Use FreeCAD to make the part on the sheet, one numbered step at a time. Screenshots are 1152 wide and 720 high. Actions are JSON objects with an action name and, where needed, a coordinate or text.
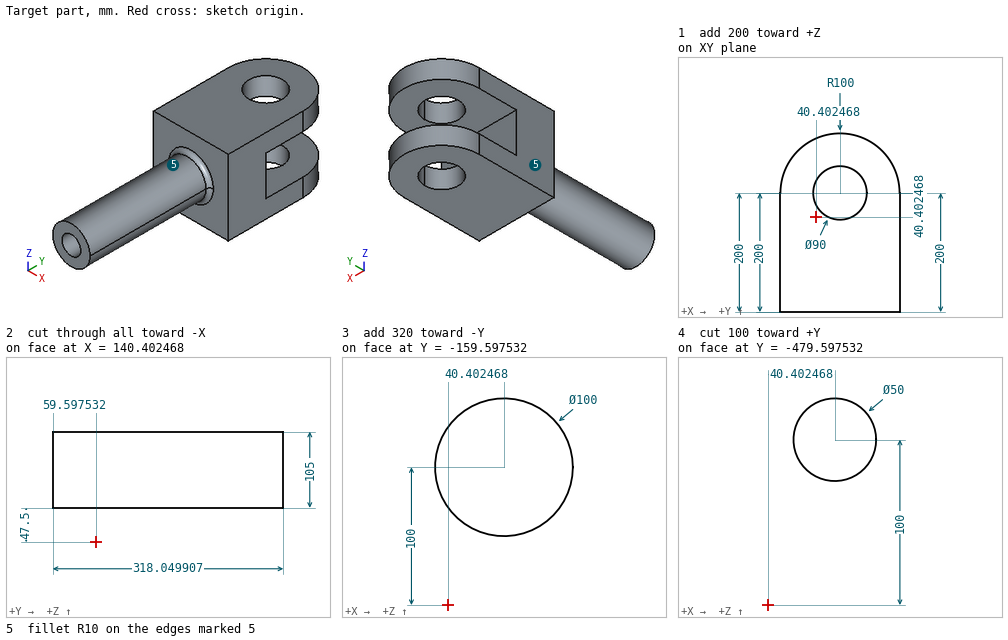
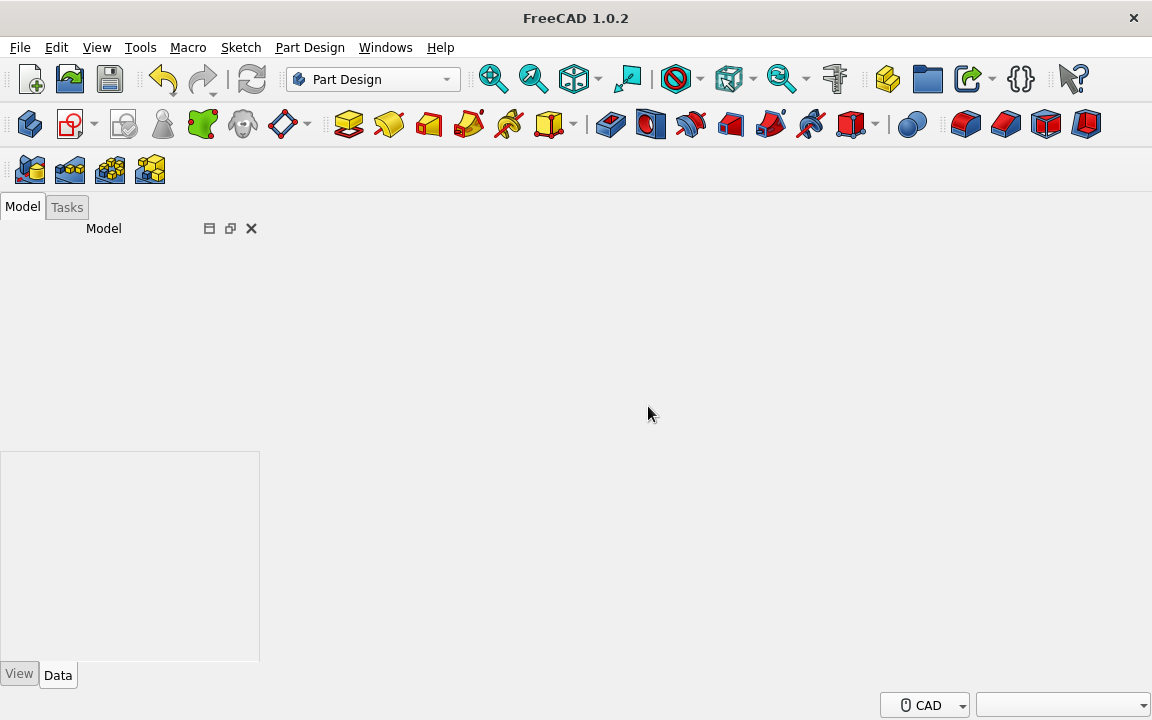
{"action": "key", "text": "ctrl+n"}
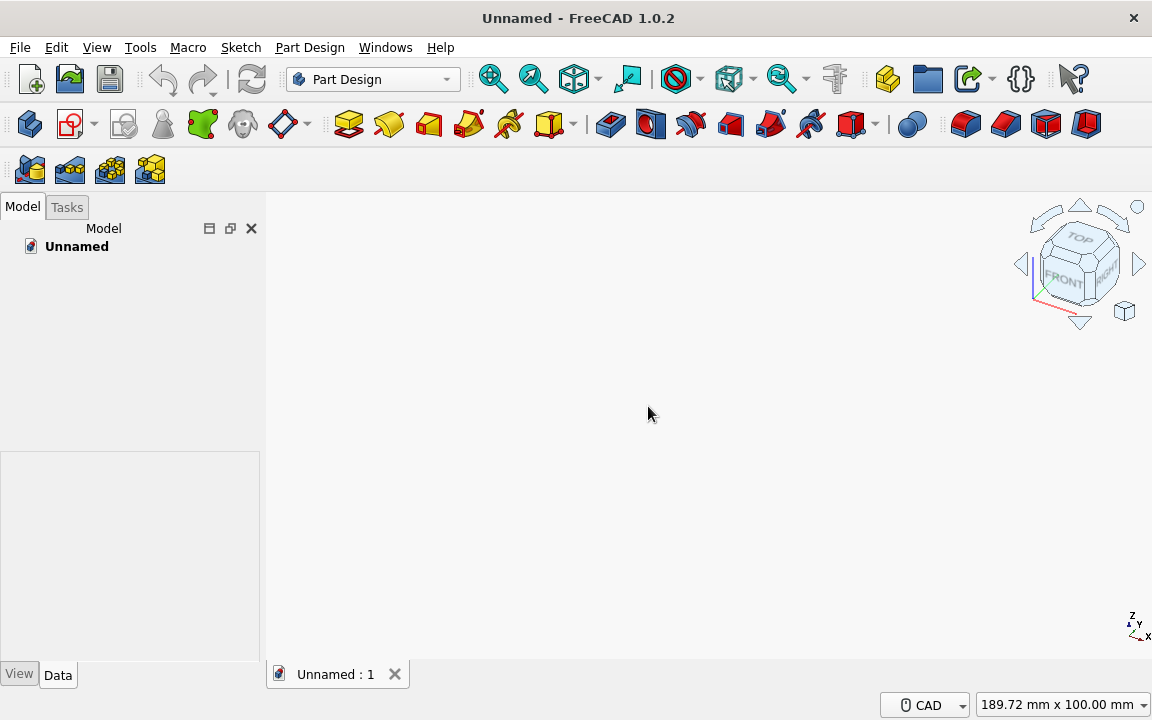
{"action": "left_click", "coordinate": [70, 124]}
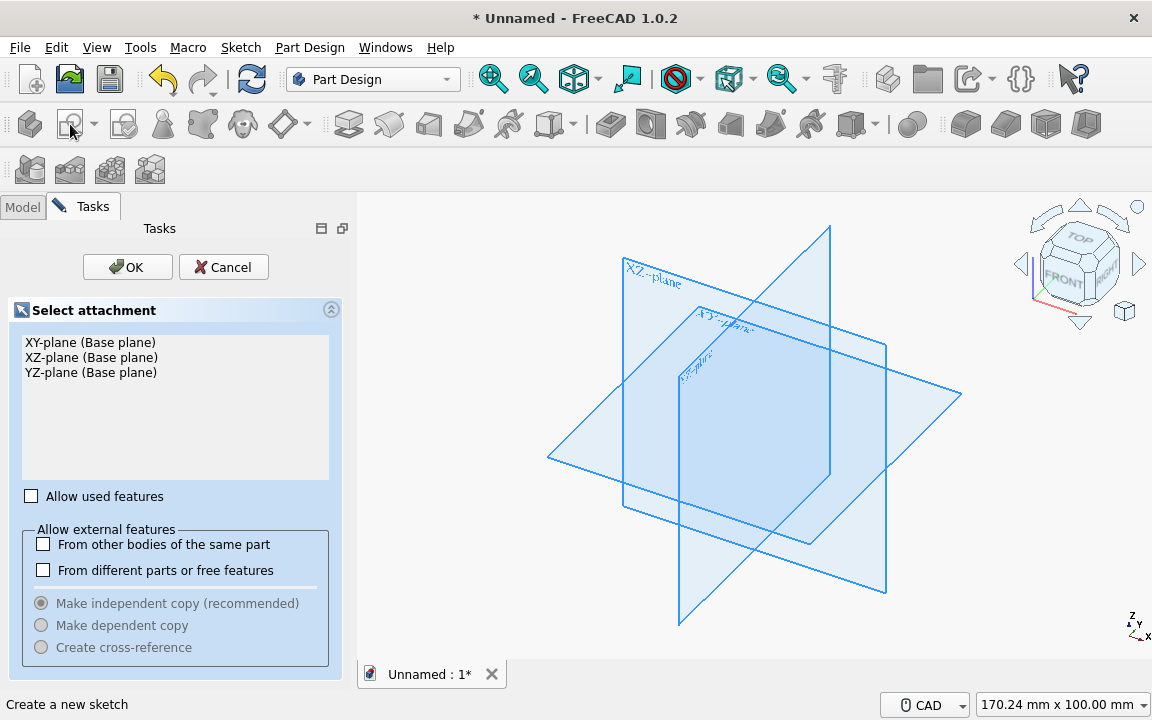
{"action": "left_click", "coordinate": [82, 342]}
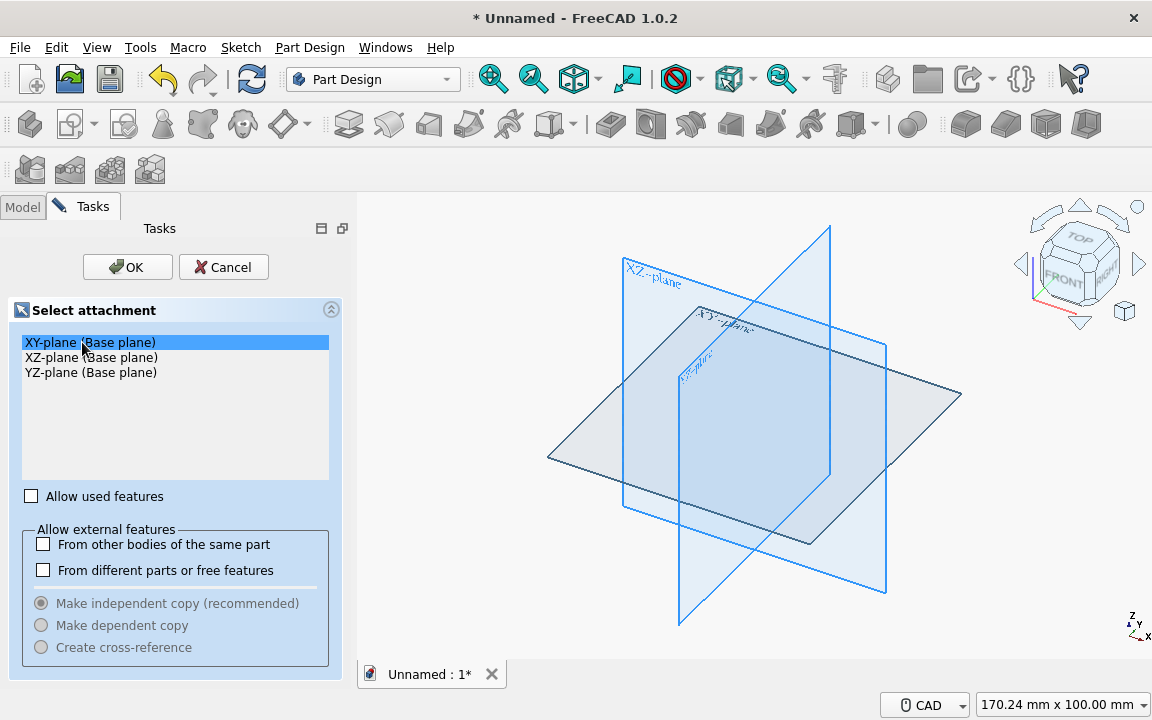
{"action": "left_click", "coordinate": [128, 267]}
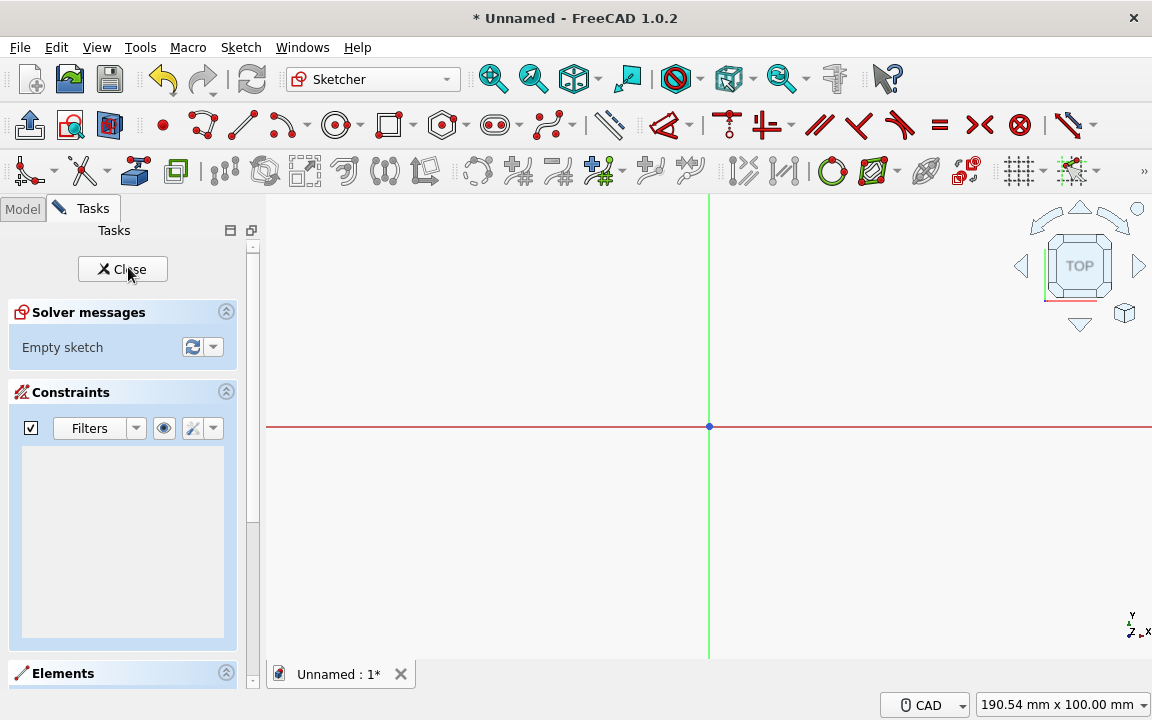
{"action": "scroll", "coordinate": [576, 415], "scroll_direction": "down", "scroll_amount": 8}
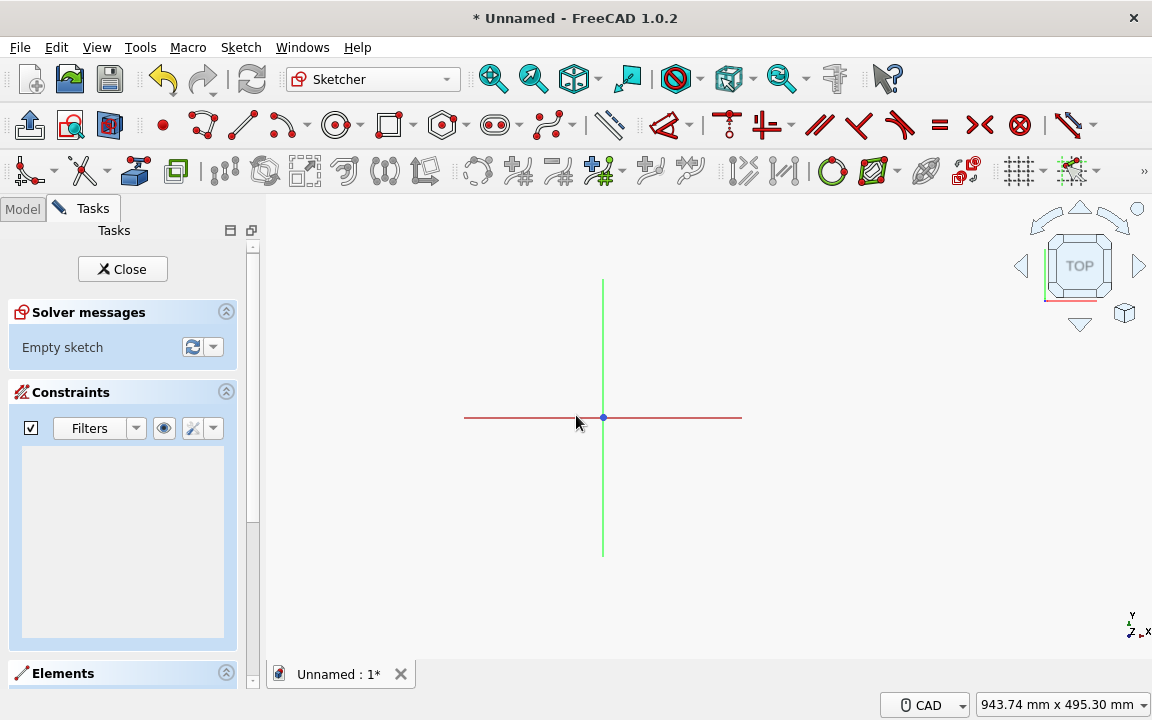
{"action": "key", "text": "g m"}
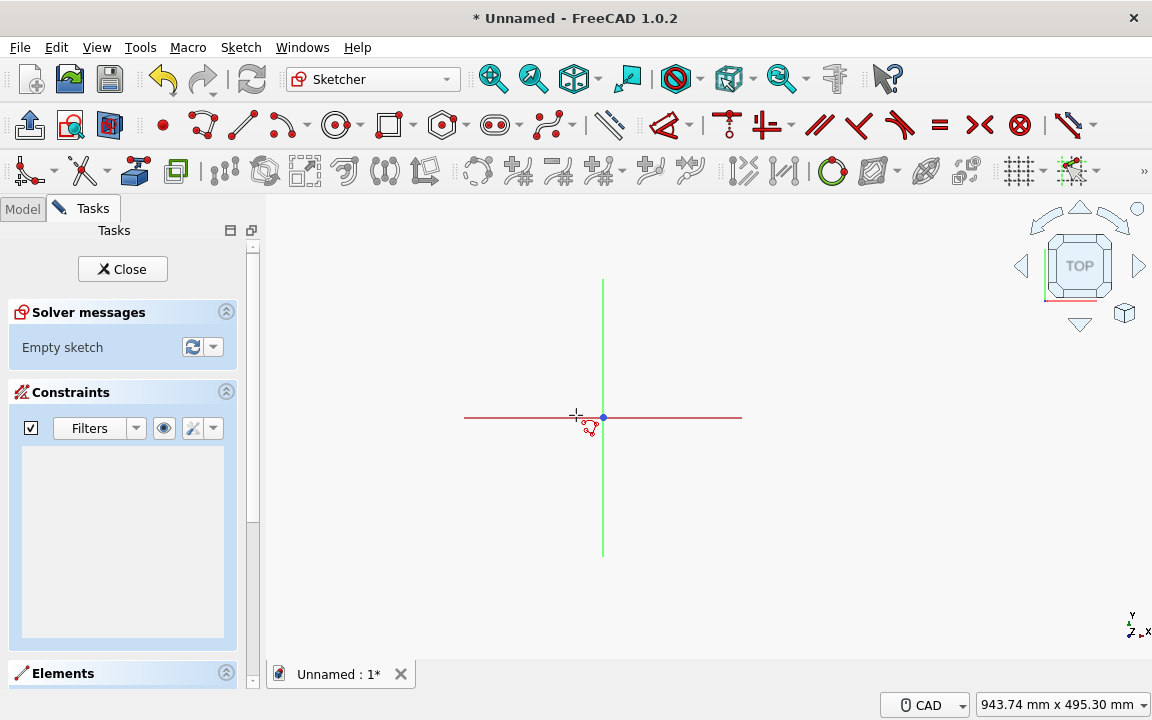
{"action": "left_click", "coordinate": [547, 380]}
{"action": "left_click", "coordinate": [547, 568]}
{"action": "left_click", "coordinate": [735, 568]}
{"action": "left_click", "coordinate": [735, 380]}
{"action": "right_click", "coordinate": [735, 380]}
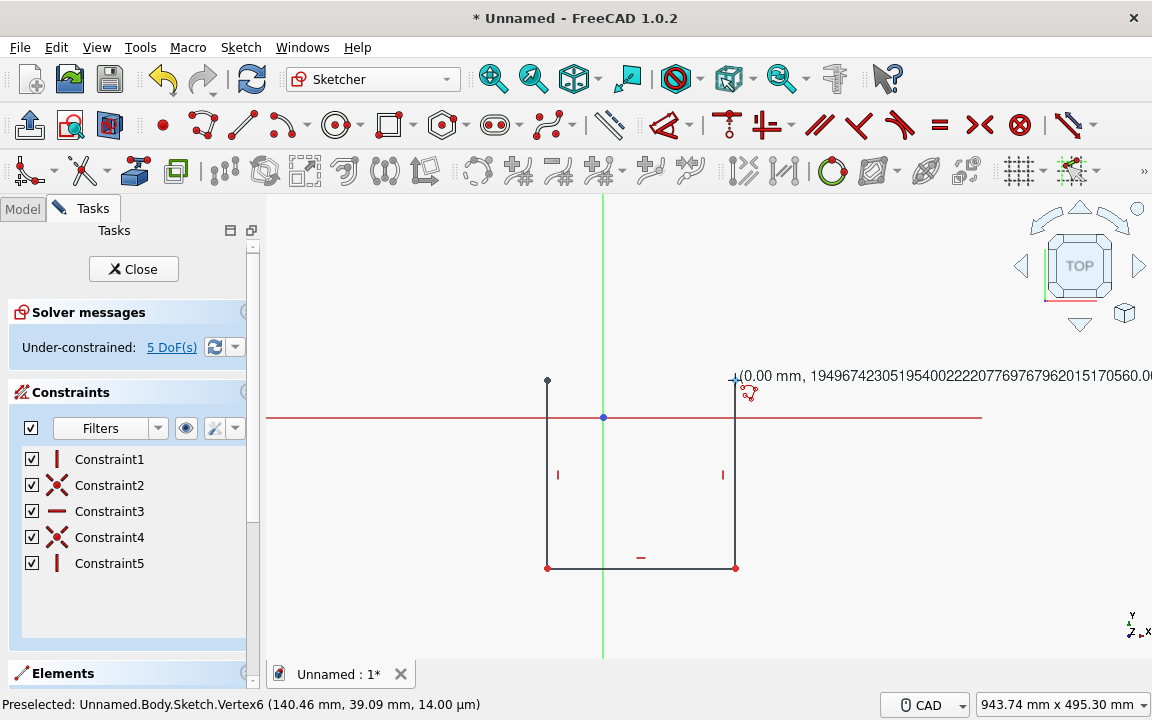
{"action": "key", "text": "g 3 a"}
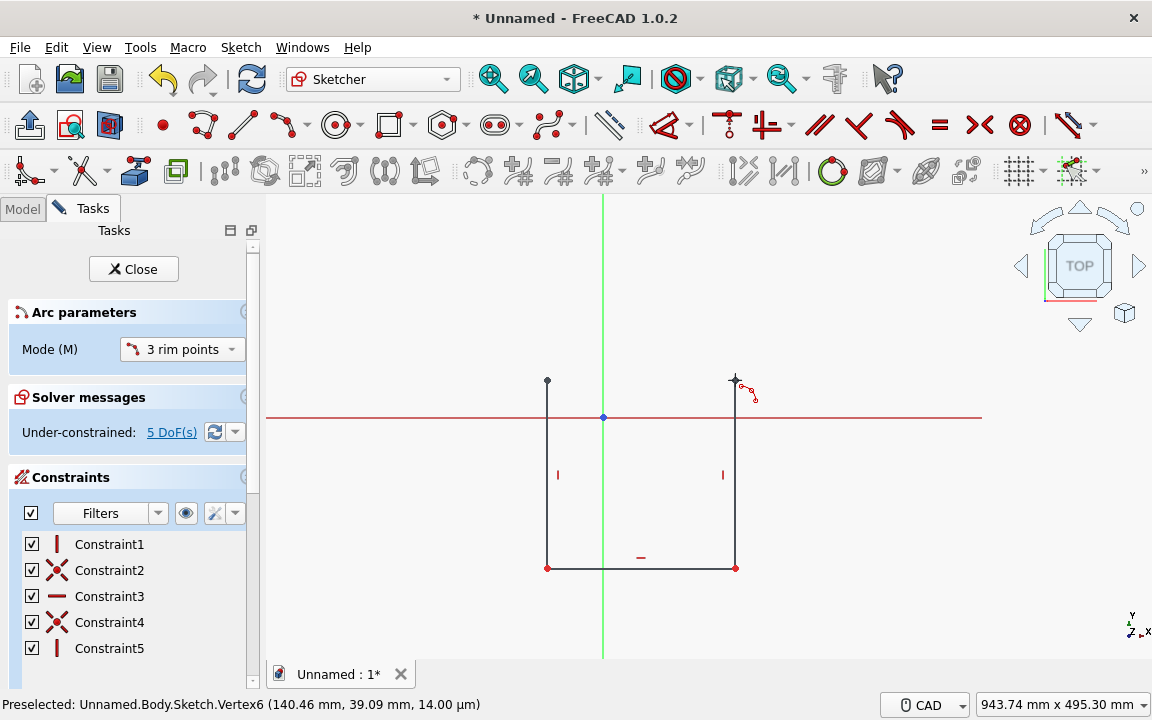
{"action": "left_click", "coordinate": [735, 381]}
{"action": "left_click", "coordinate": [547, 381]}
{"action": "left_click", "coordinate": [641, 286]}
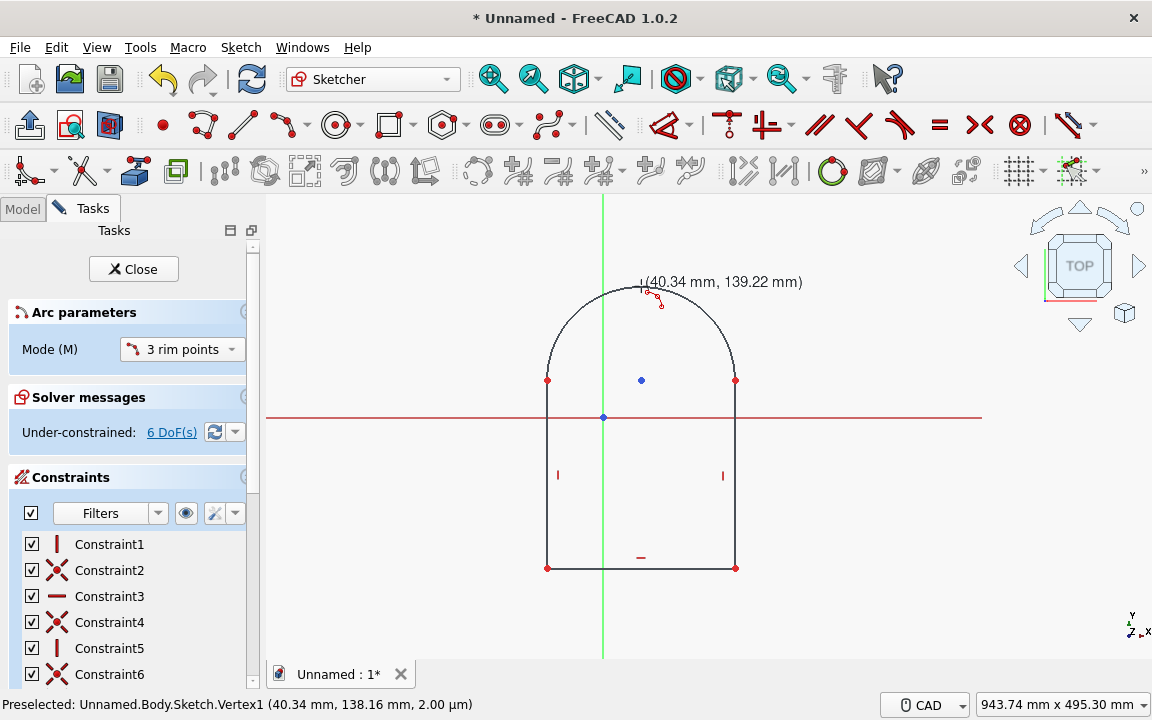
{"action": "key", "text": "g c"}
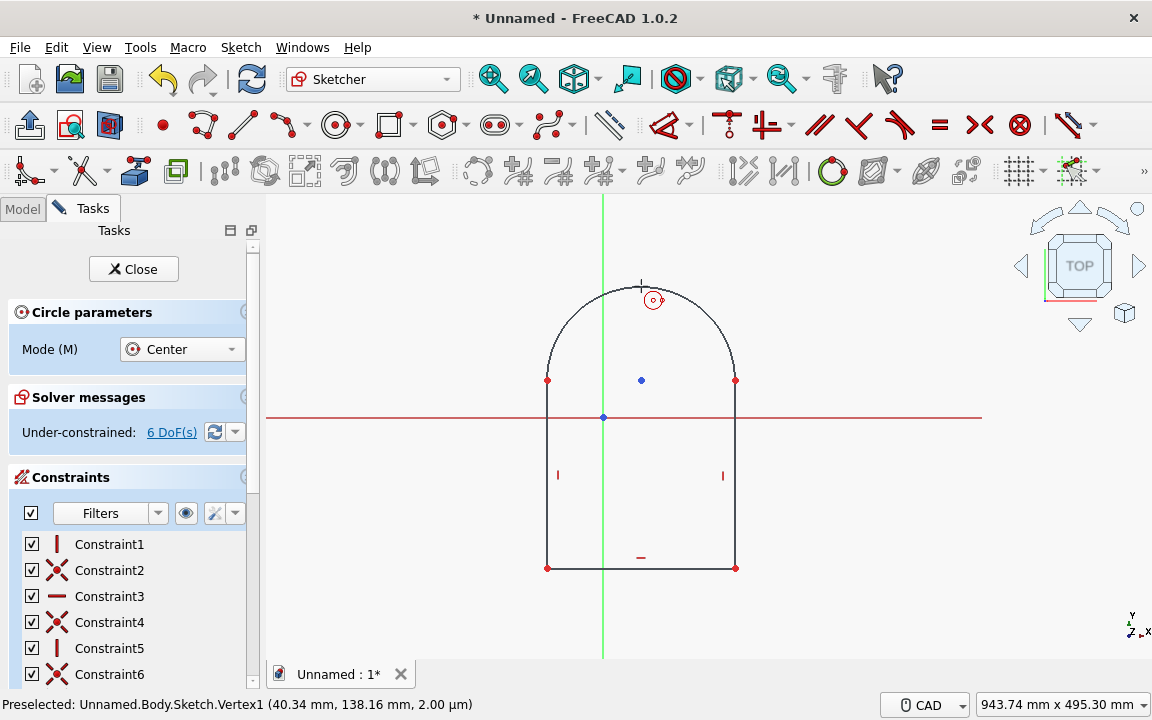
{"action": "left_click", "coordinate": [641, 380]}
{"action": "mouse_move", "coordinate": [671, 350]}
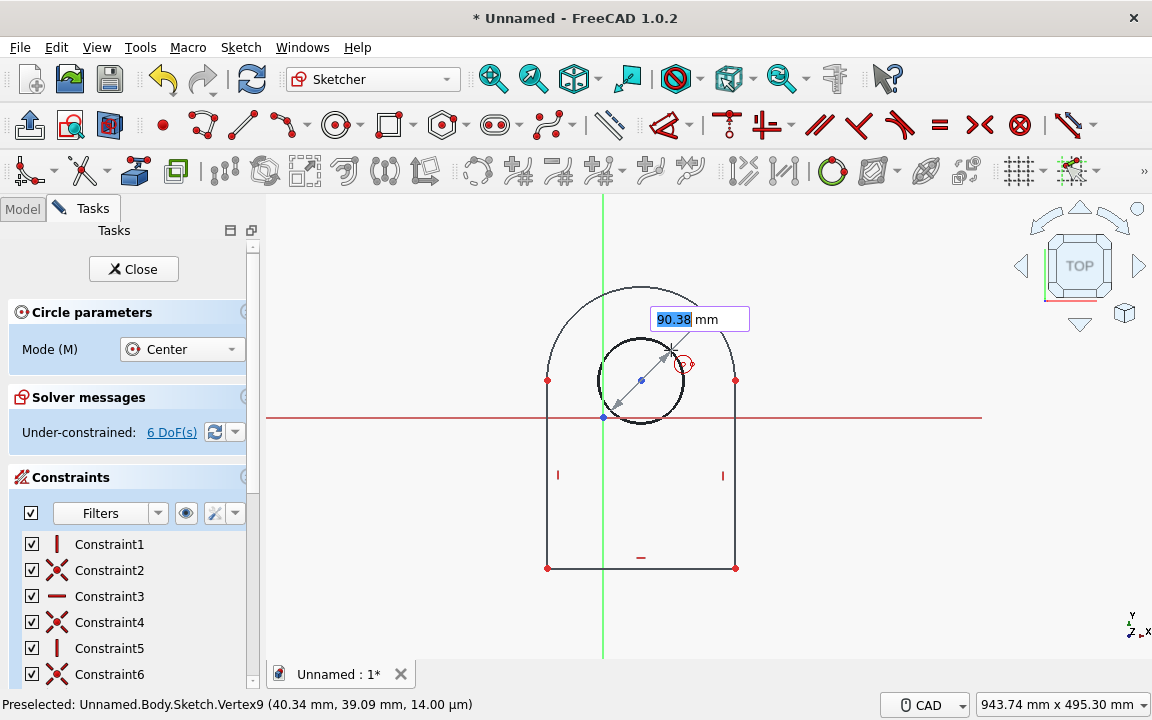
{"action": "type", "text": "90"}
{"action": "key", "text": "Return"}
{"action": "key", "text": "Escape"}